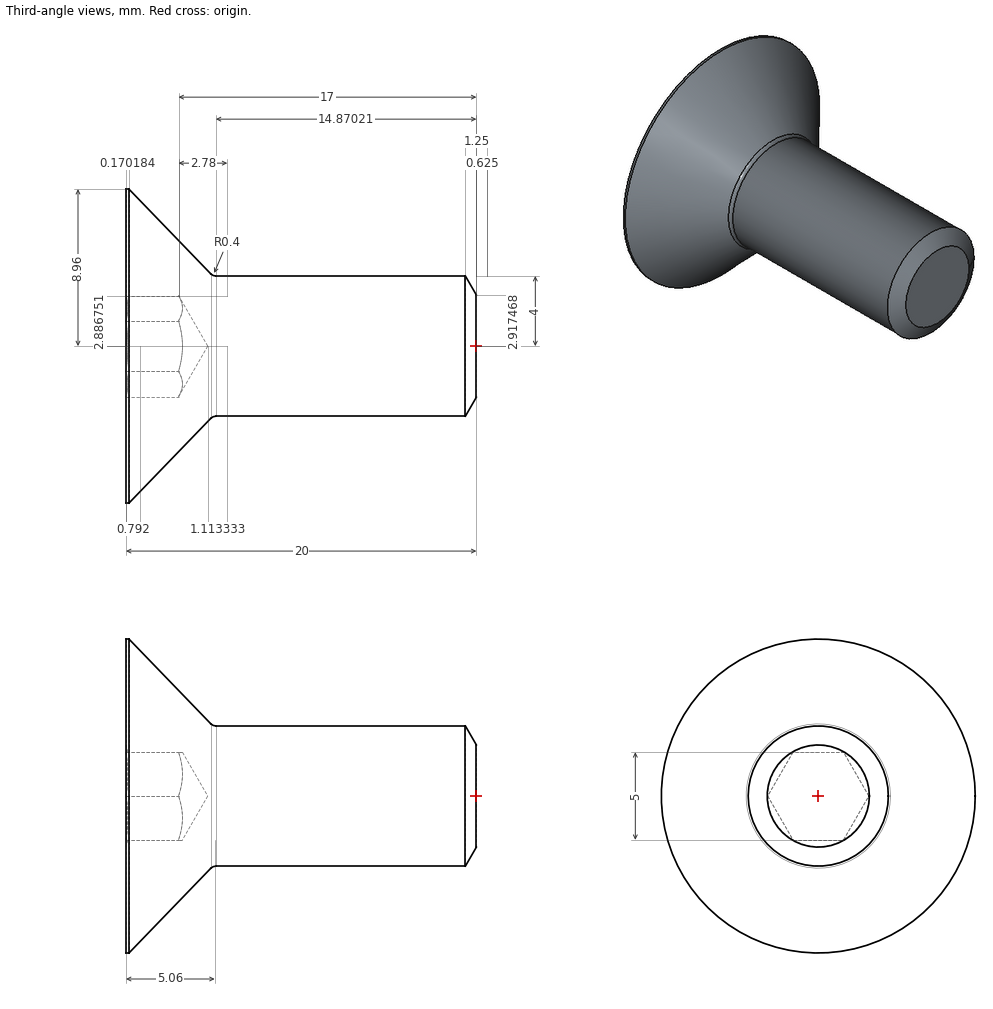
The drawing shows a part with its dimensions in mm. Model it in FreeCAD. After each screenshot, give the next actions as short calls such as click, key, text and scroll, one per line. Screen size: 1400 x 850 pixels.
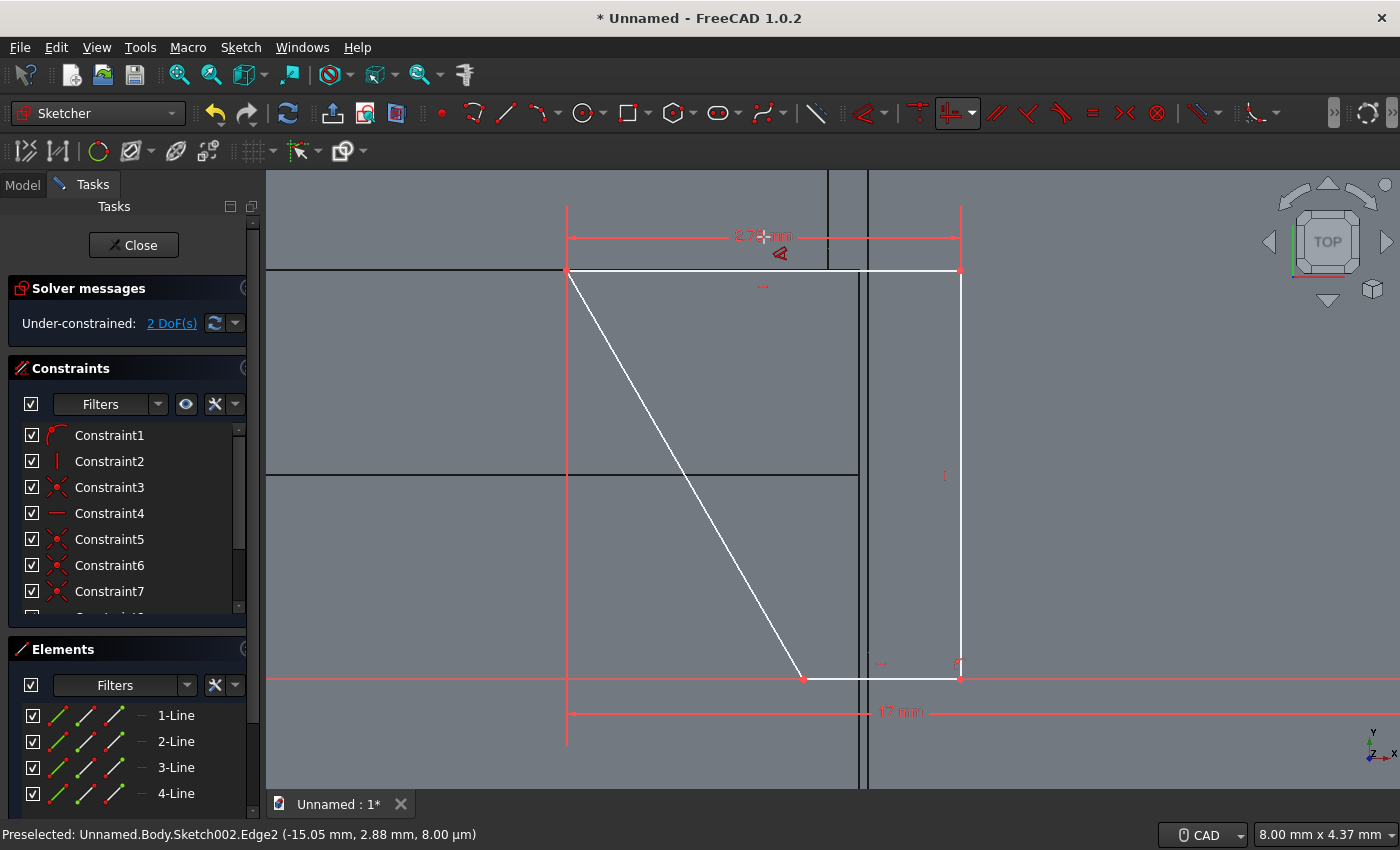
click(961, 557)
click(995, 475)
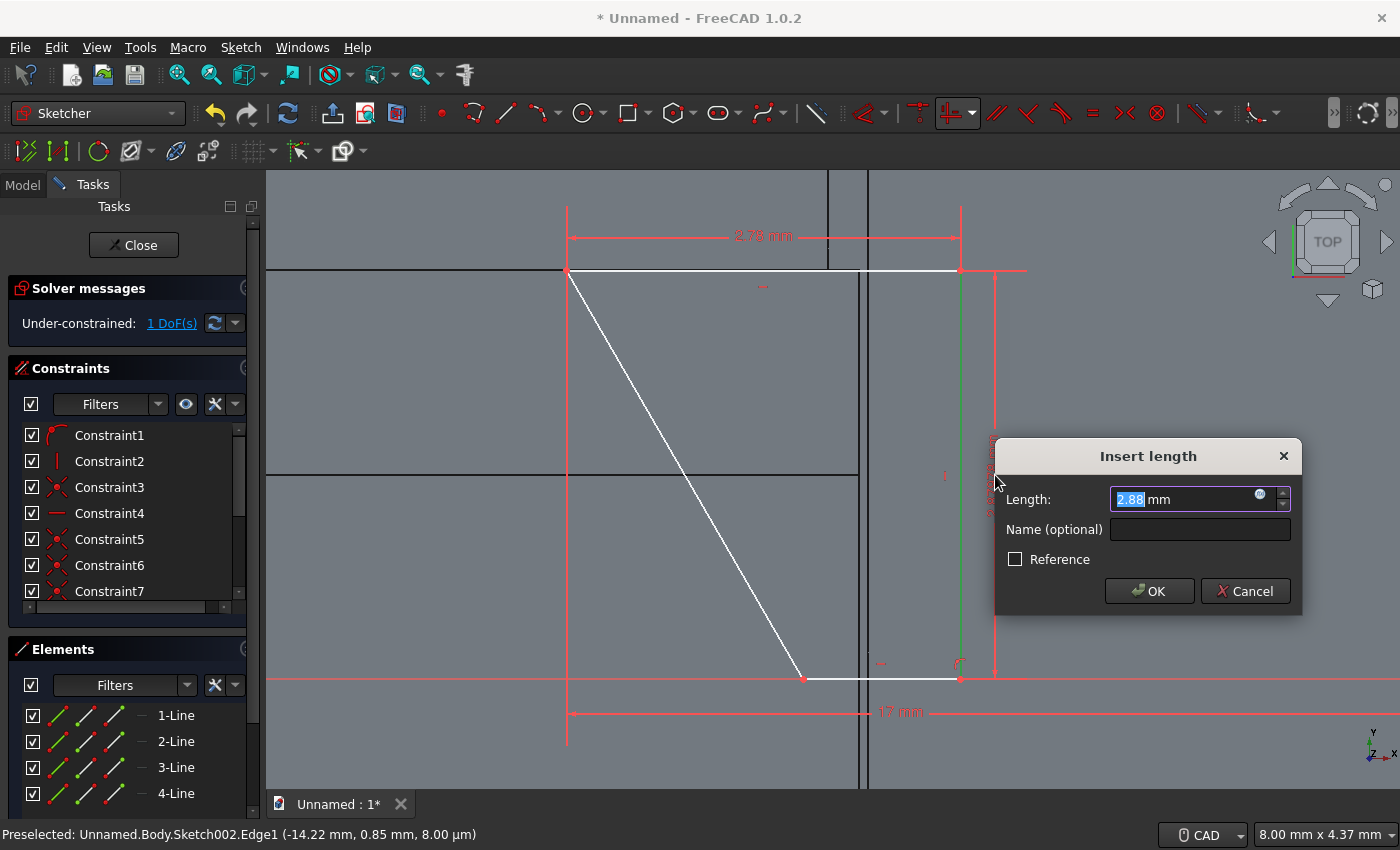
text(2.886751)
key(Return)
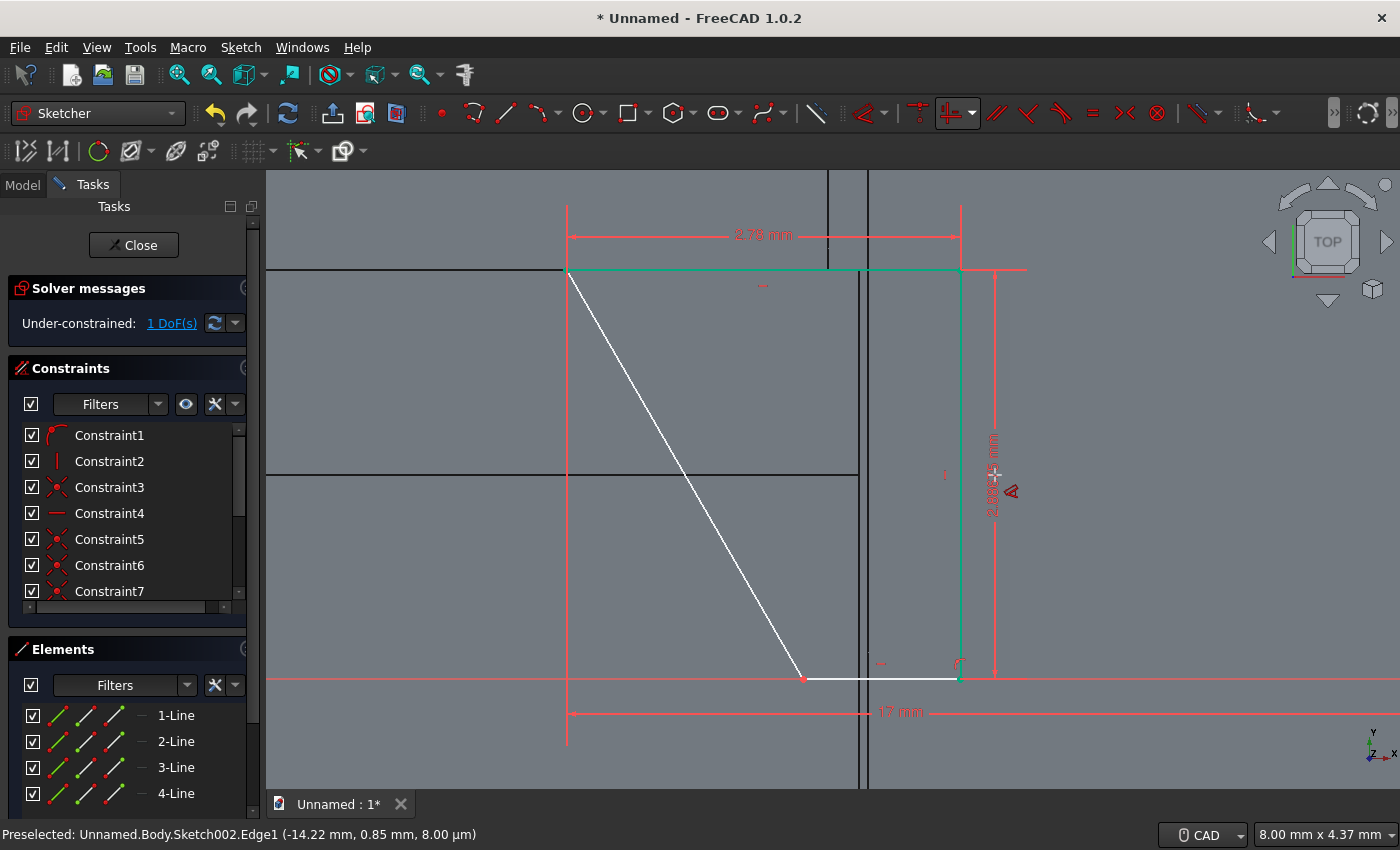
click(850, 679)
click(827, 713)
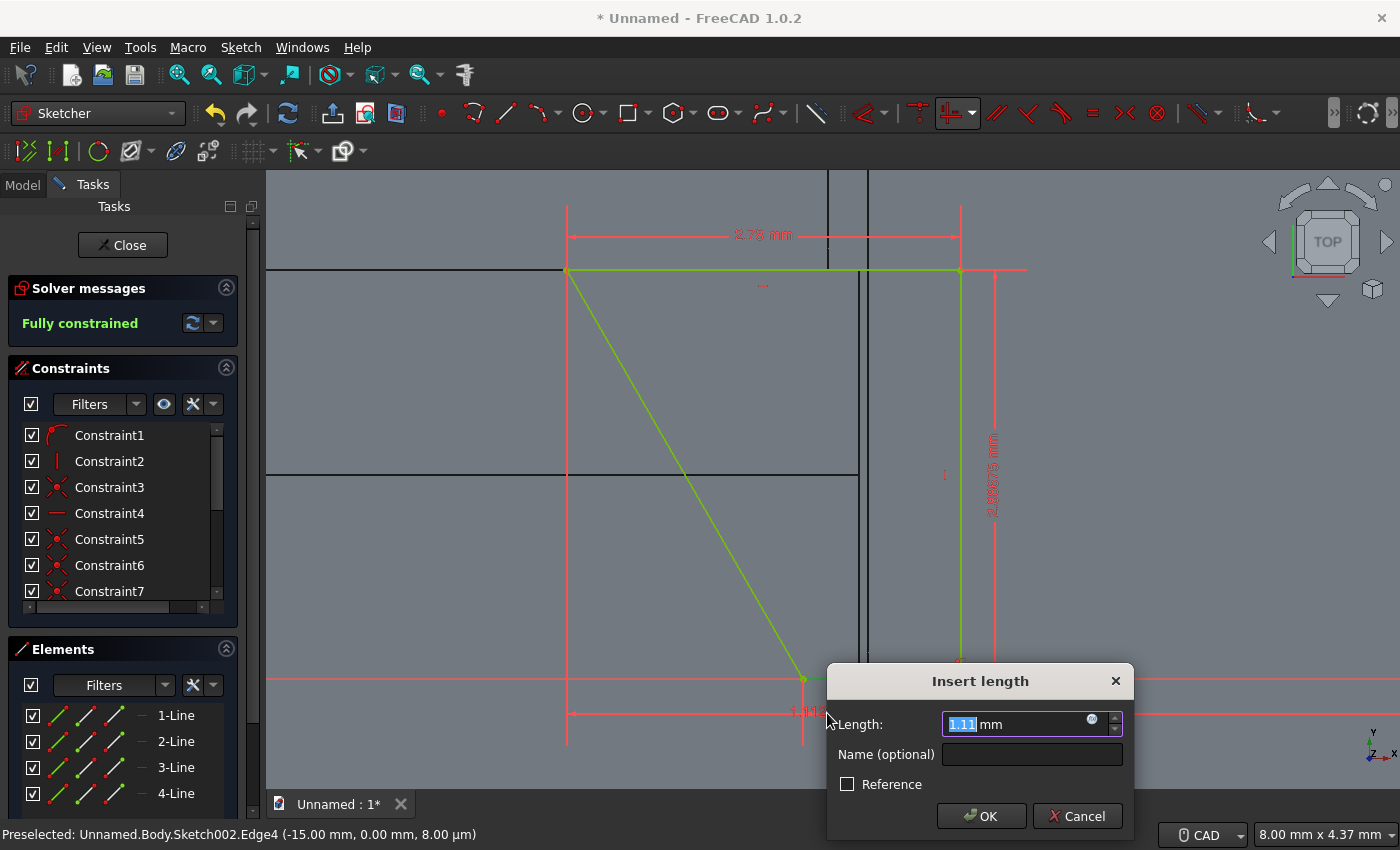
text(1.113333)
key(Return)
key(Escape)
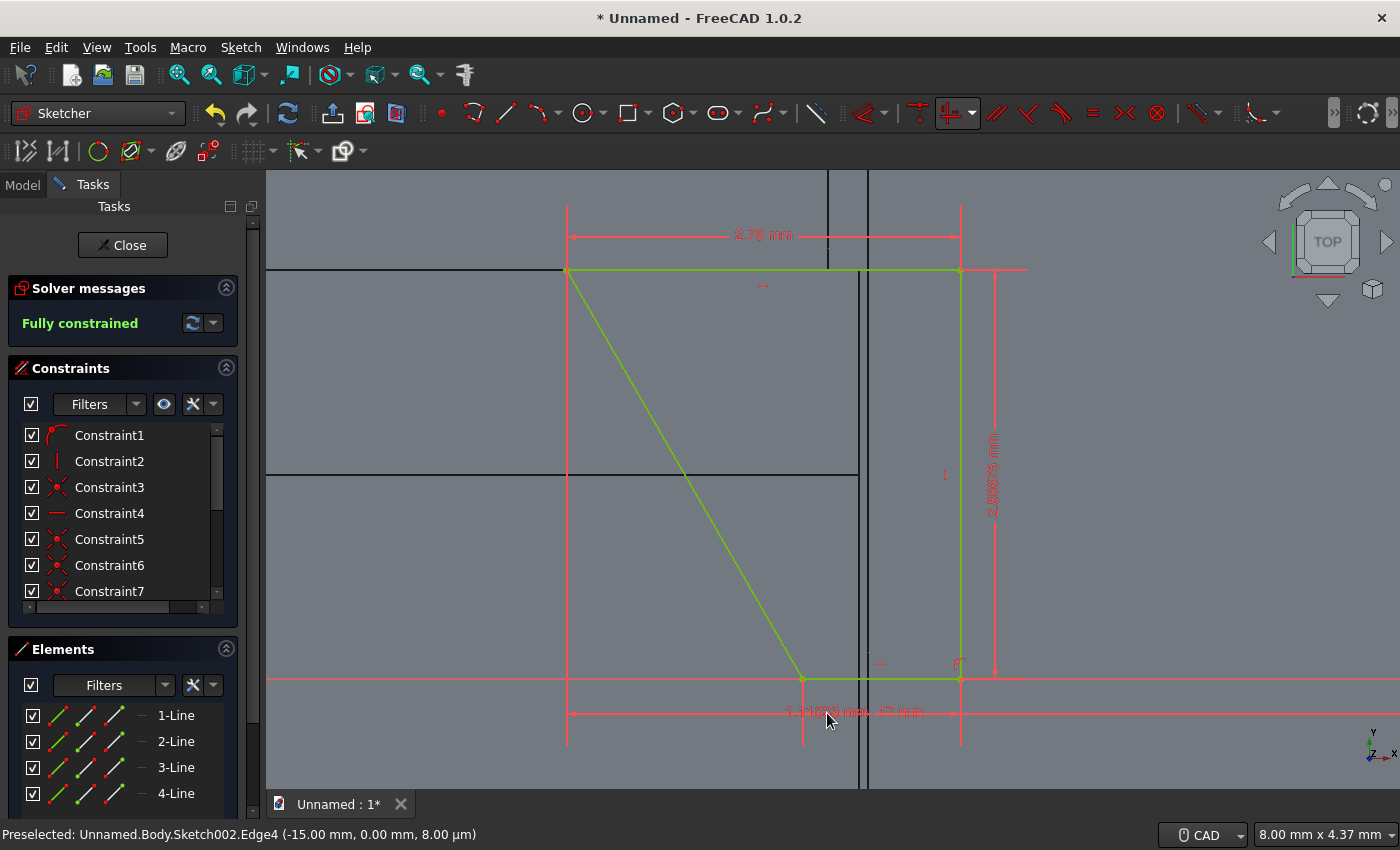
click(123, 245)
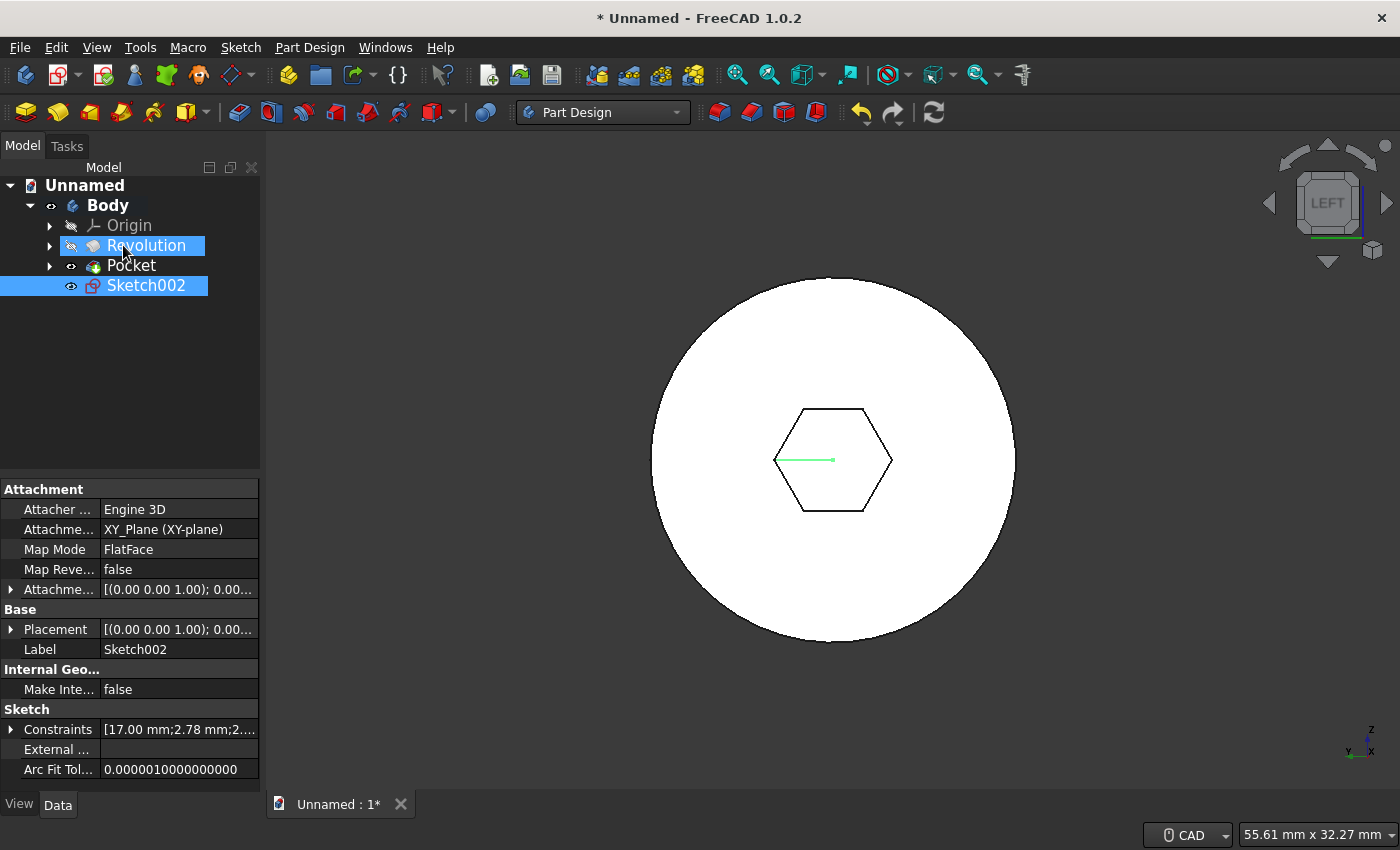
click(58, 112)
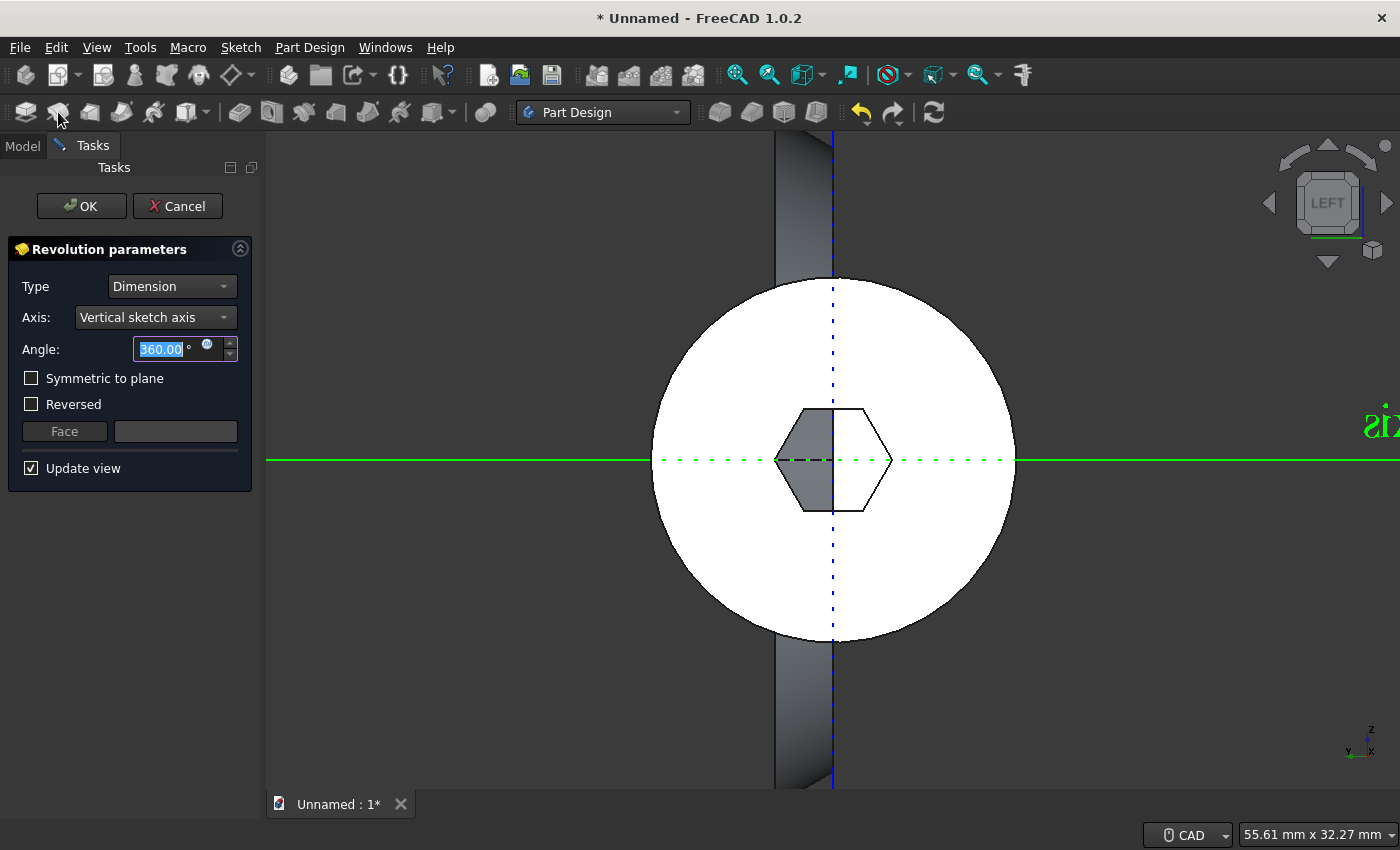
click(156, 318)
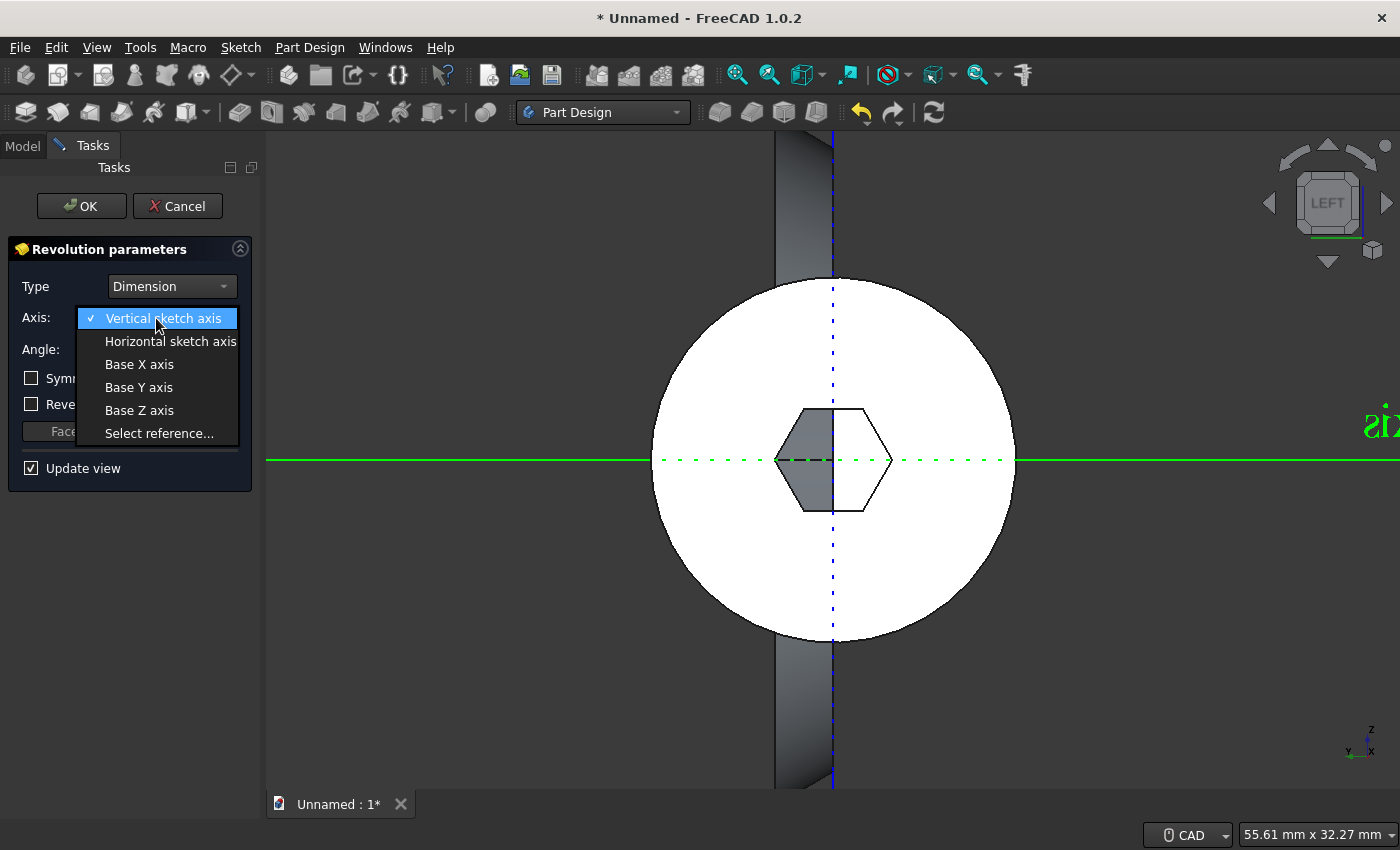
click(156, 342)